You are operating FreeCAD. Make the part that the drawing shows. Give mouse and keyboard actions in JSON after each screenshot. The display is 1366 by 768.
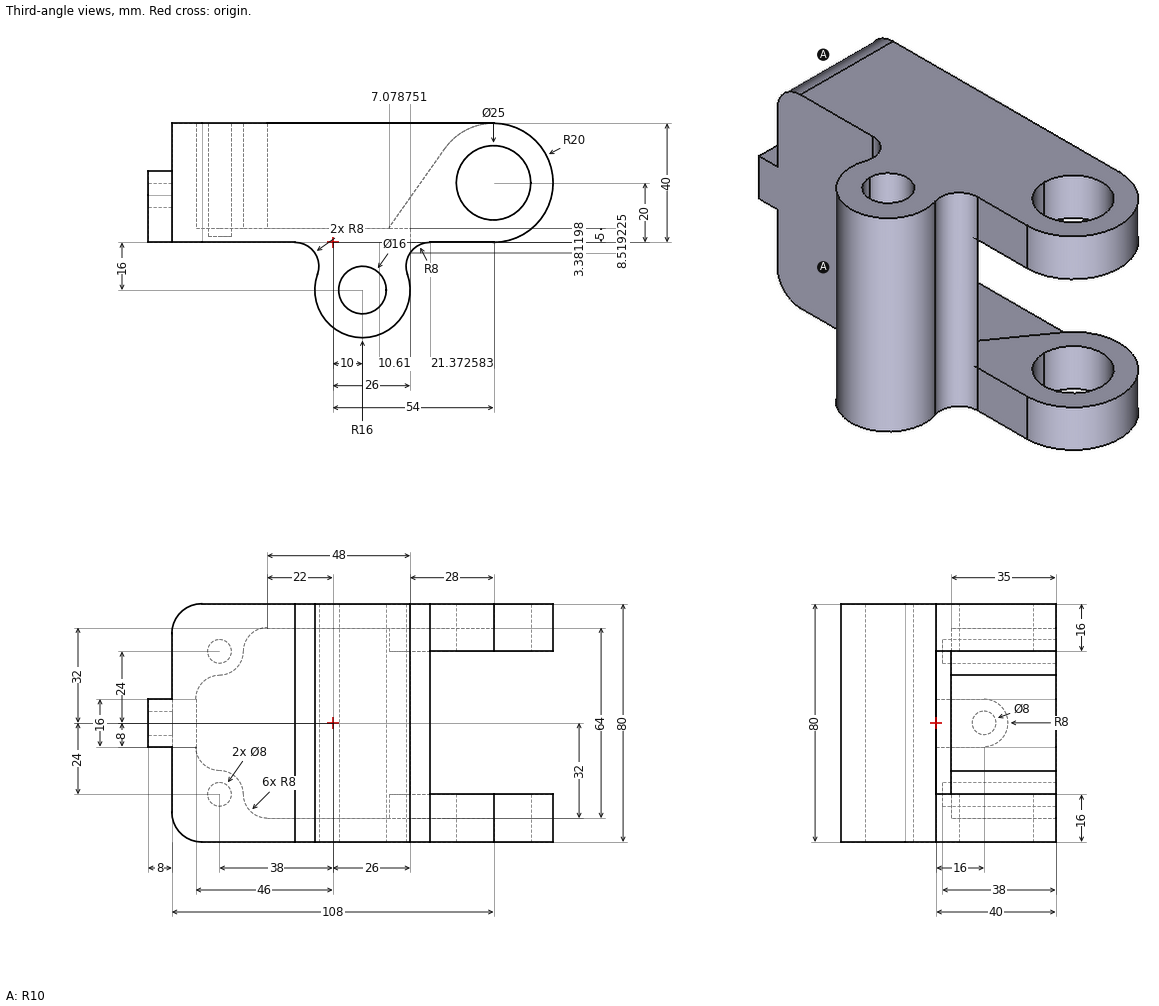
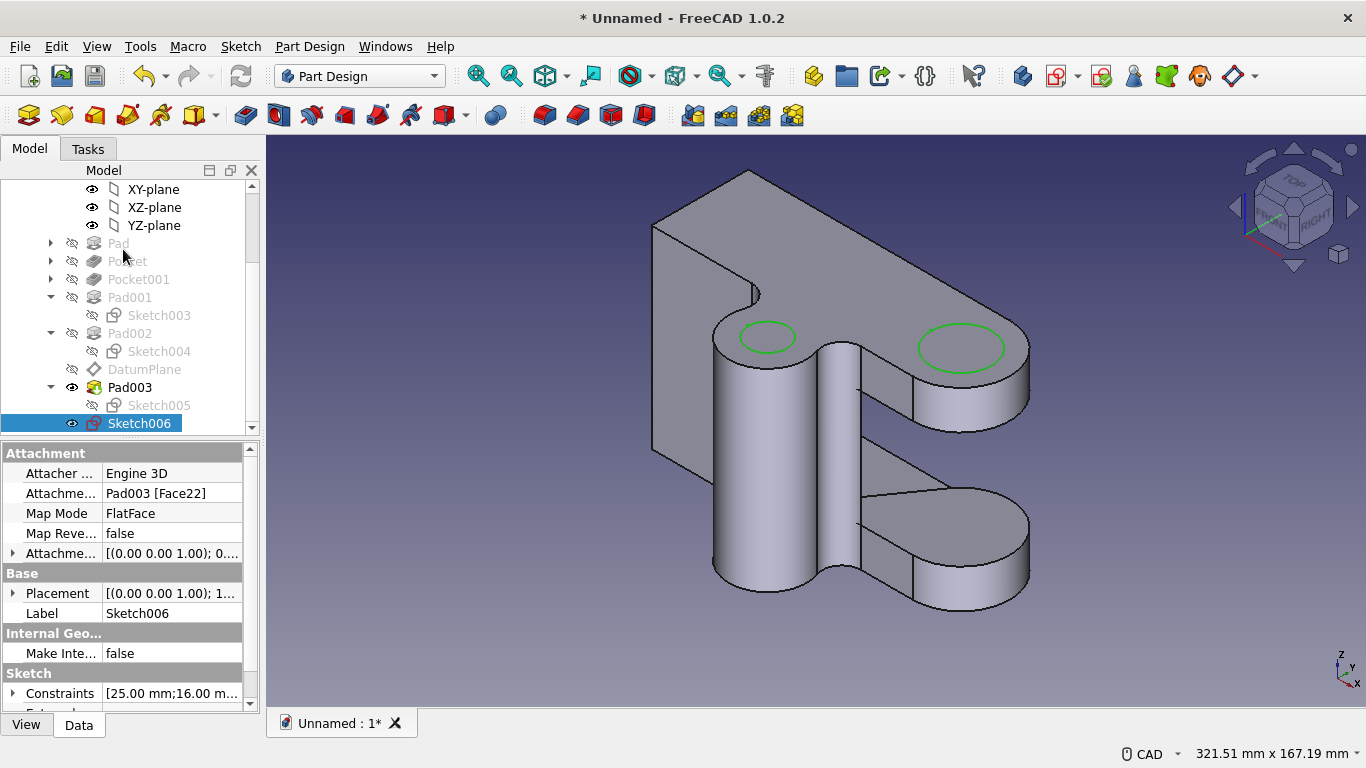
{"action": "left_click", "coordinate": [246, 116]}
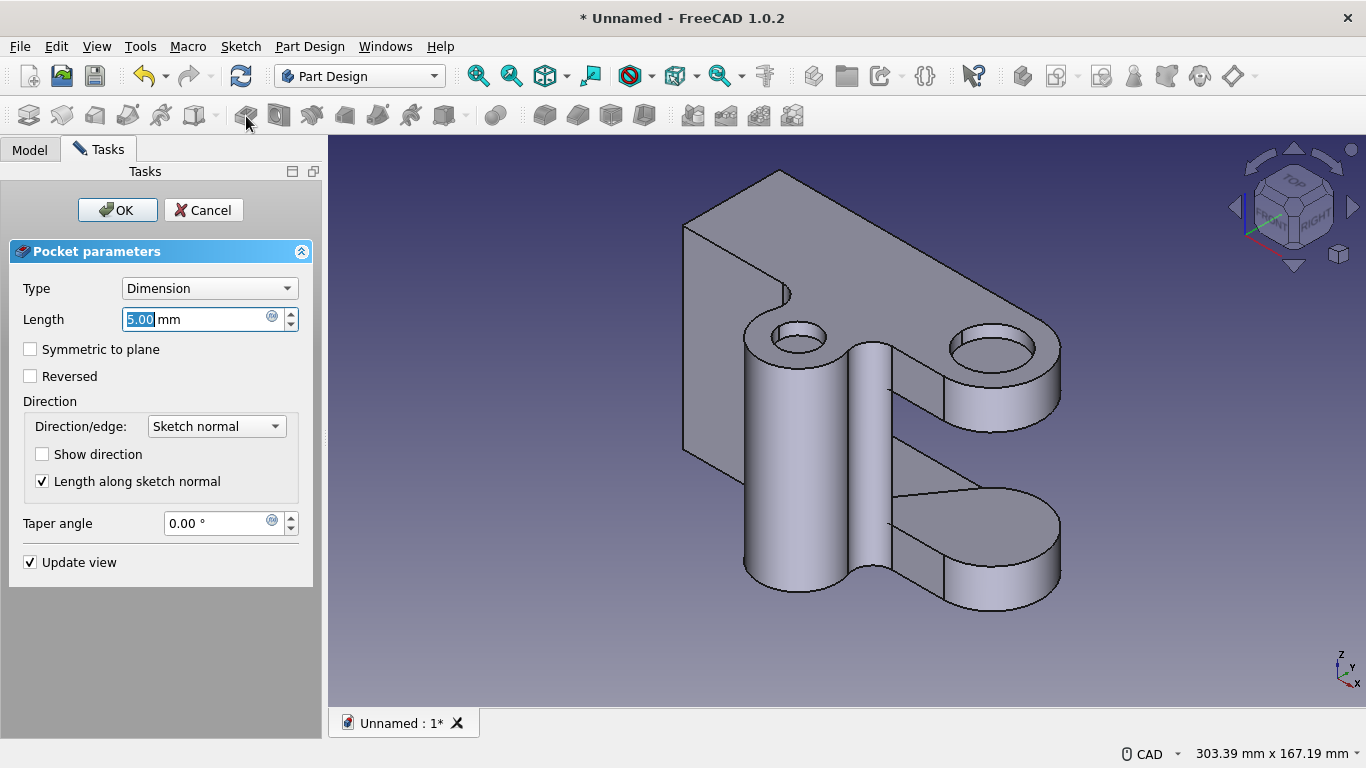
{"action": "left_click", "coordinate": [210, 288]}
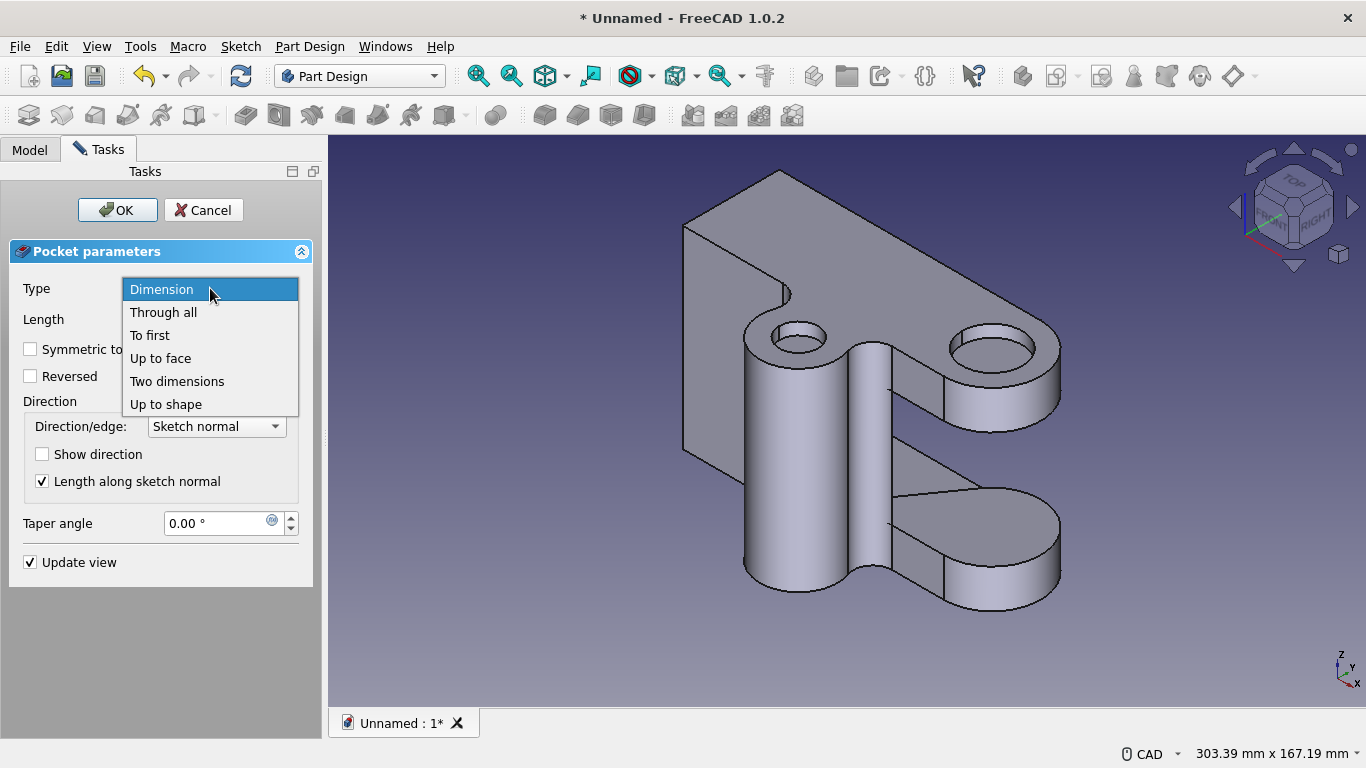
{"action": "left_click", "coordinate": [208, 312]}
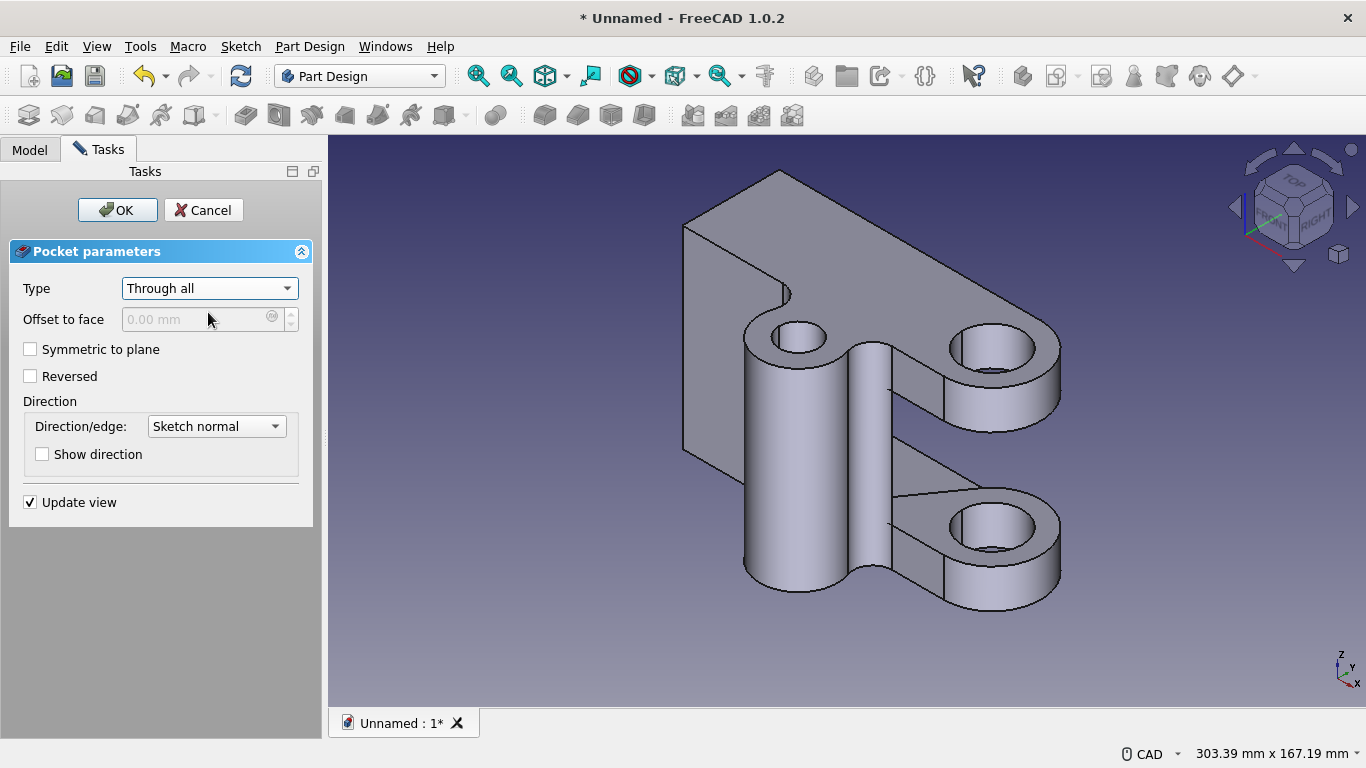
{"action": "left_click", "coordinate": [118, 210]}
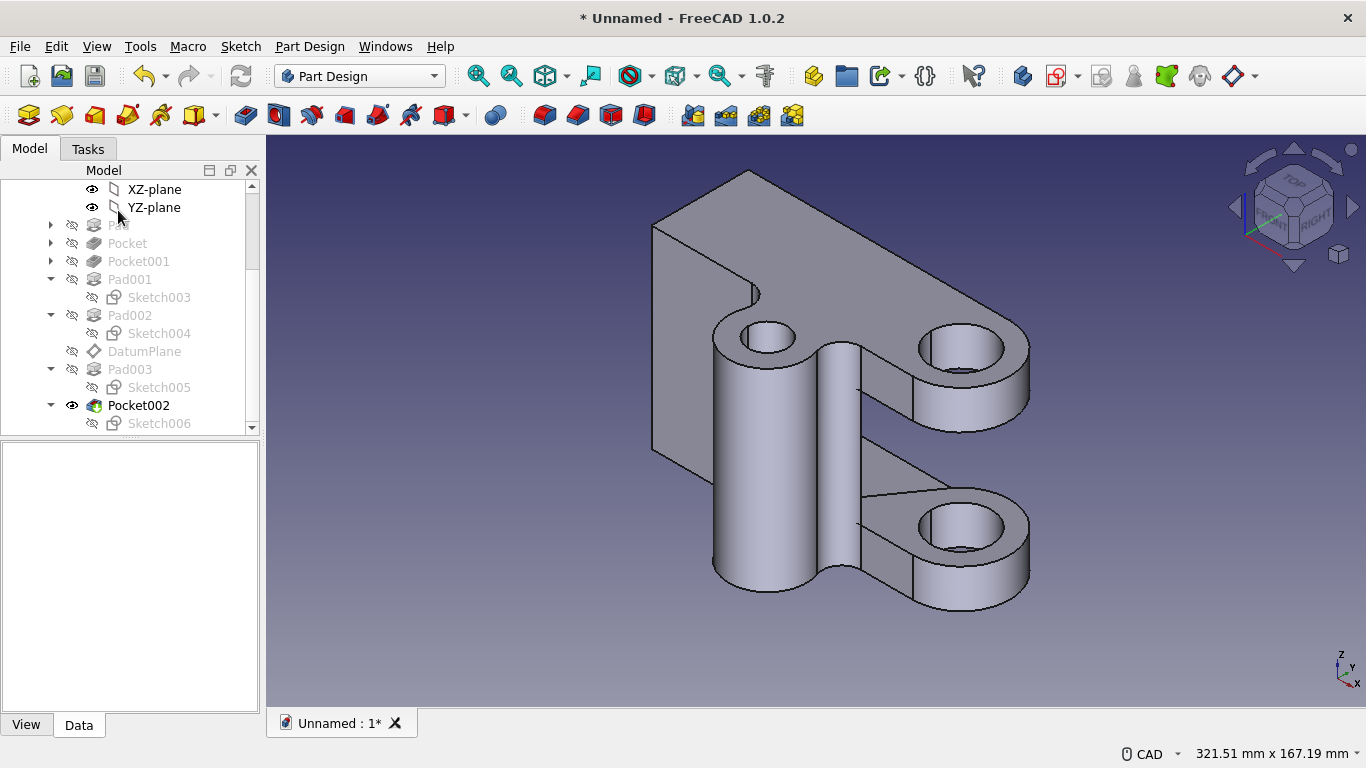
{"action": "key", "text": "4"}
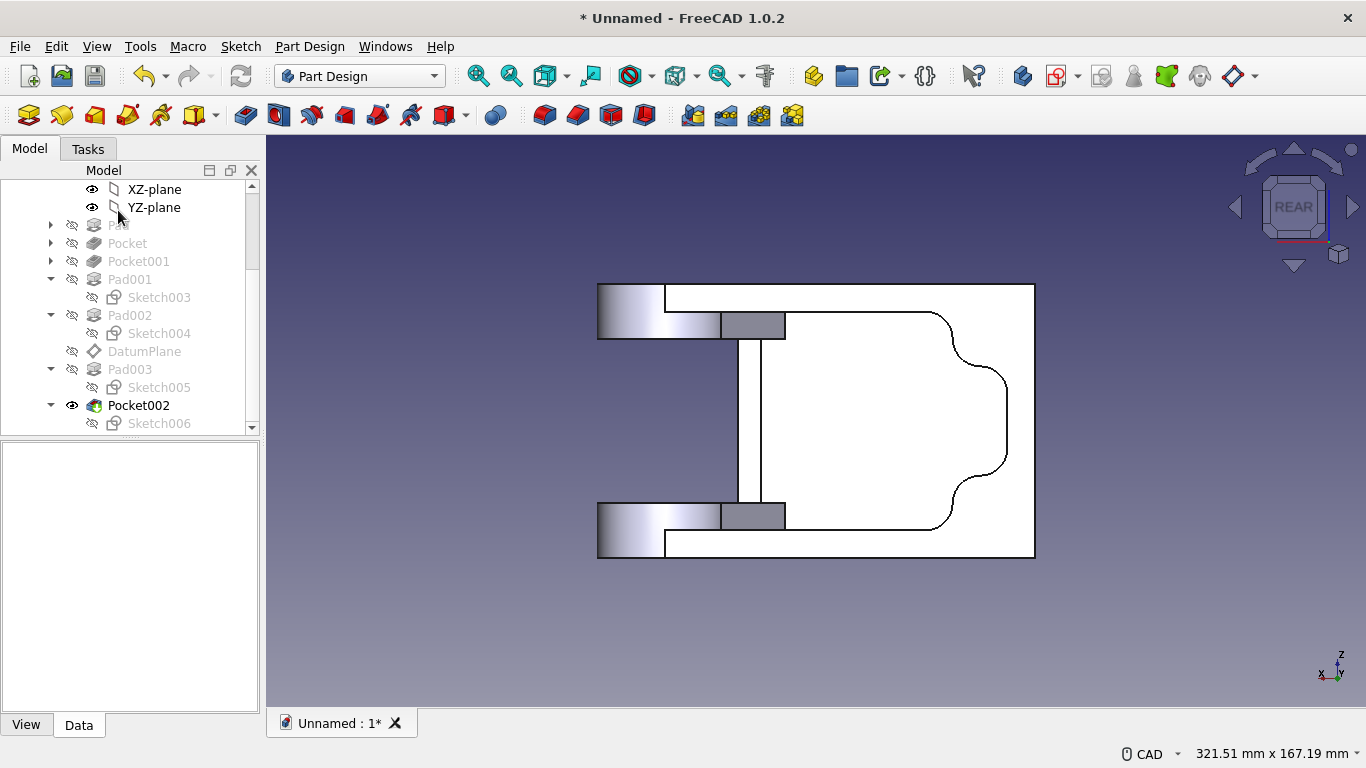
{"action": "left_click", "coordinate": [1008, 342]}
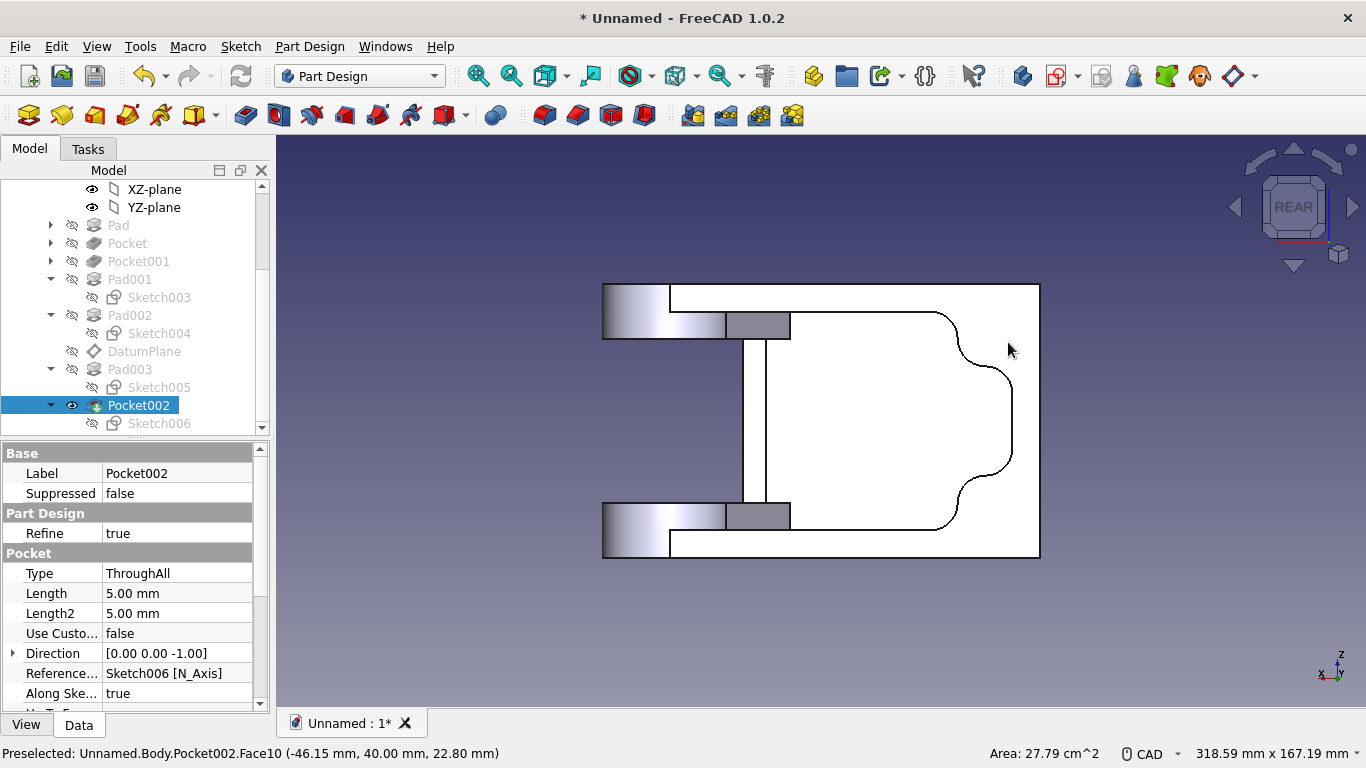
{"action": "left_click", "coordinate": [1056, 76]}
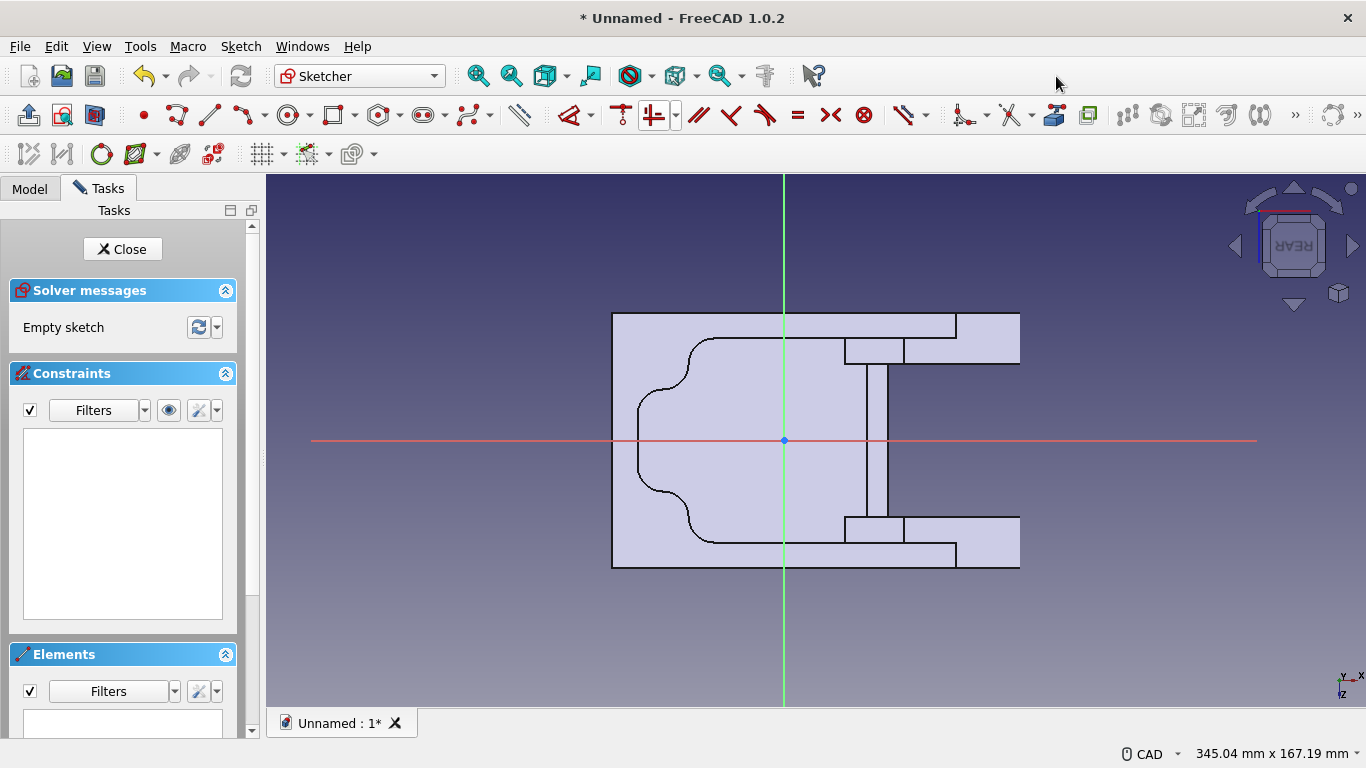
{"action": "scroll", "coordinate": [681, 441], "scroll_direction": "up", "scroll_amount": 3}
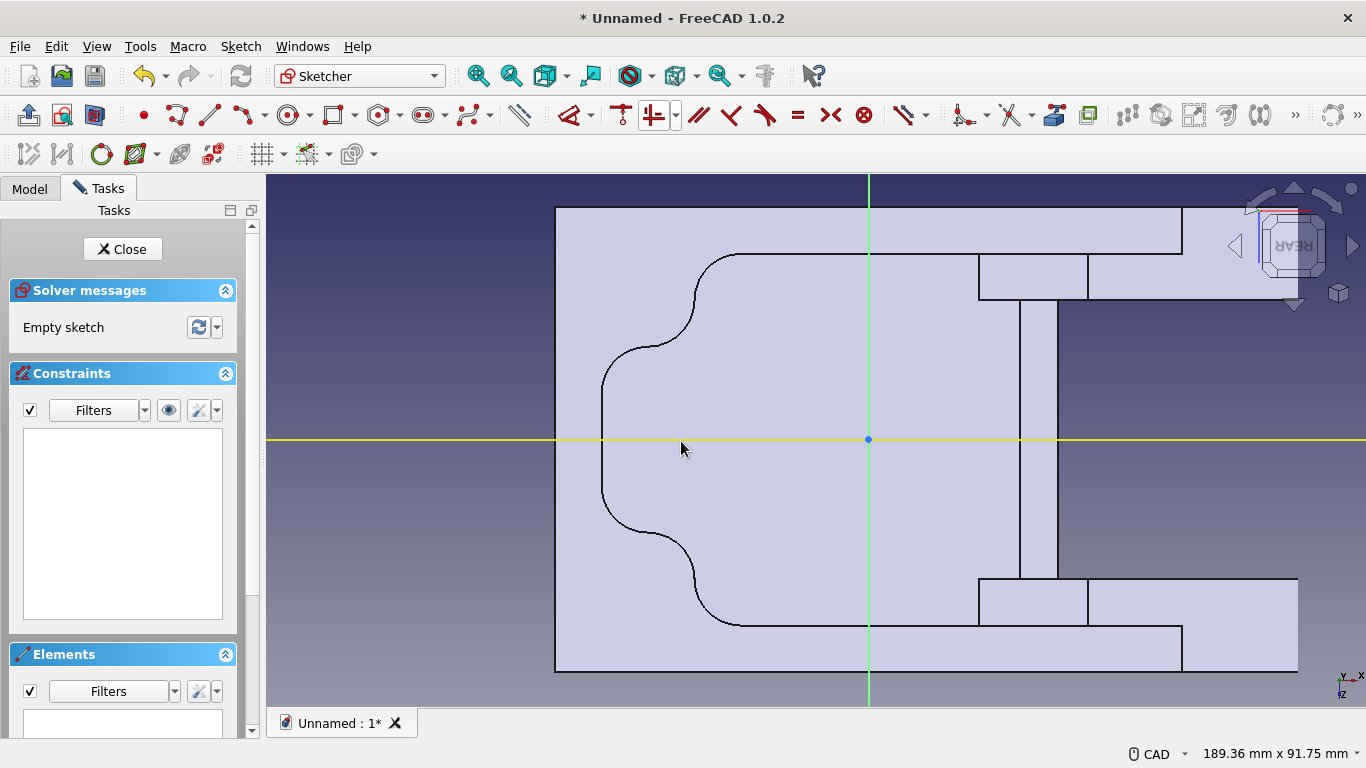
{"action": "key", "text": "g c"}